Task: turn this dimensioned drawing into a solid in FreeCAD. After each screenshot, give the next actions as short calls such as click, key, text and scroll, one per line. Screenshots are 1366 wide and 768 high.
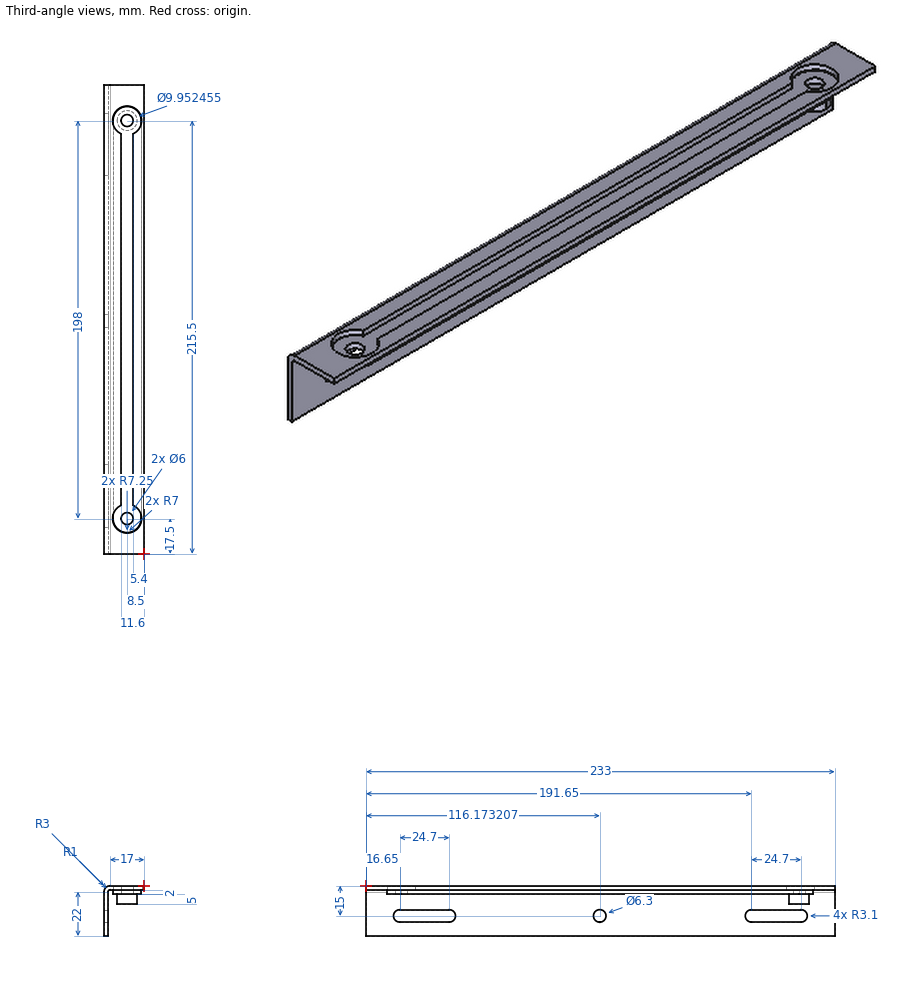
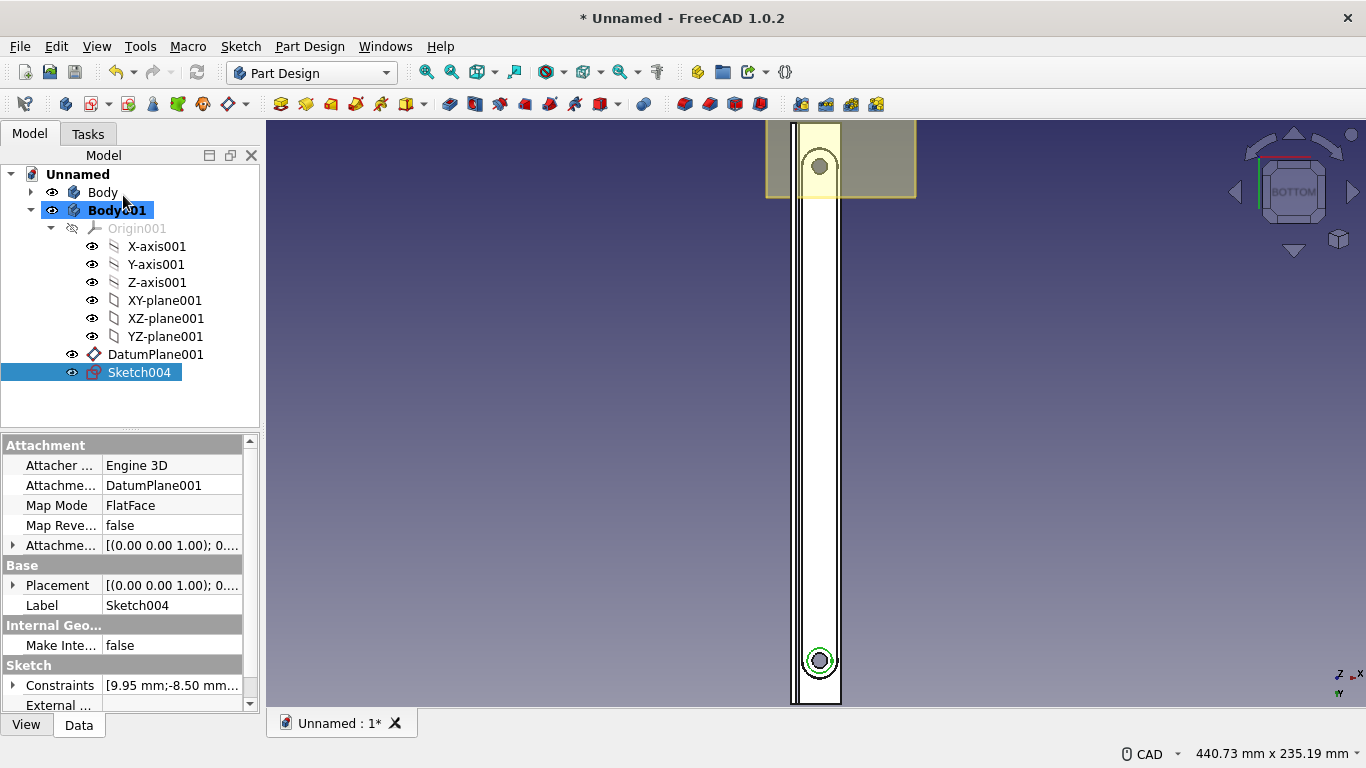
click(281, 104)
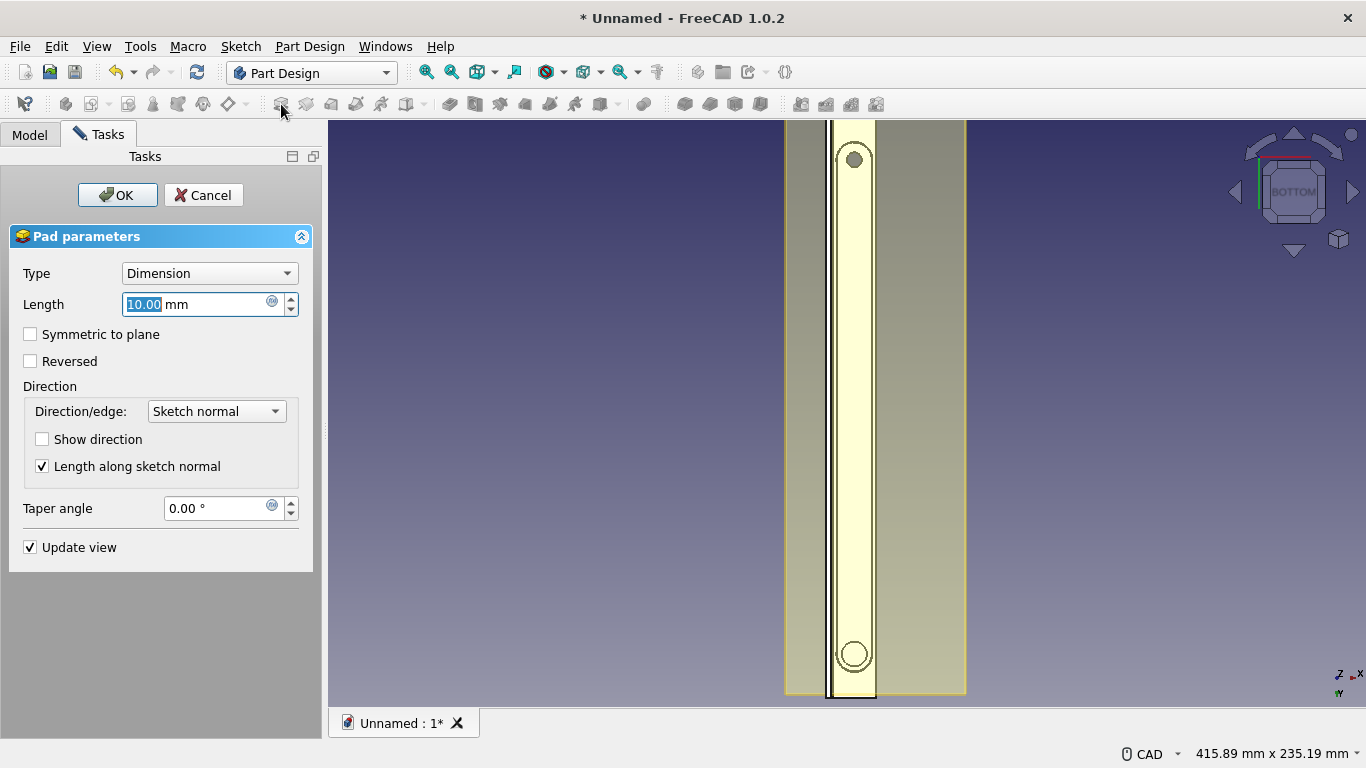
text(5)
key(Tab)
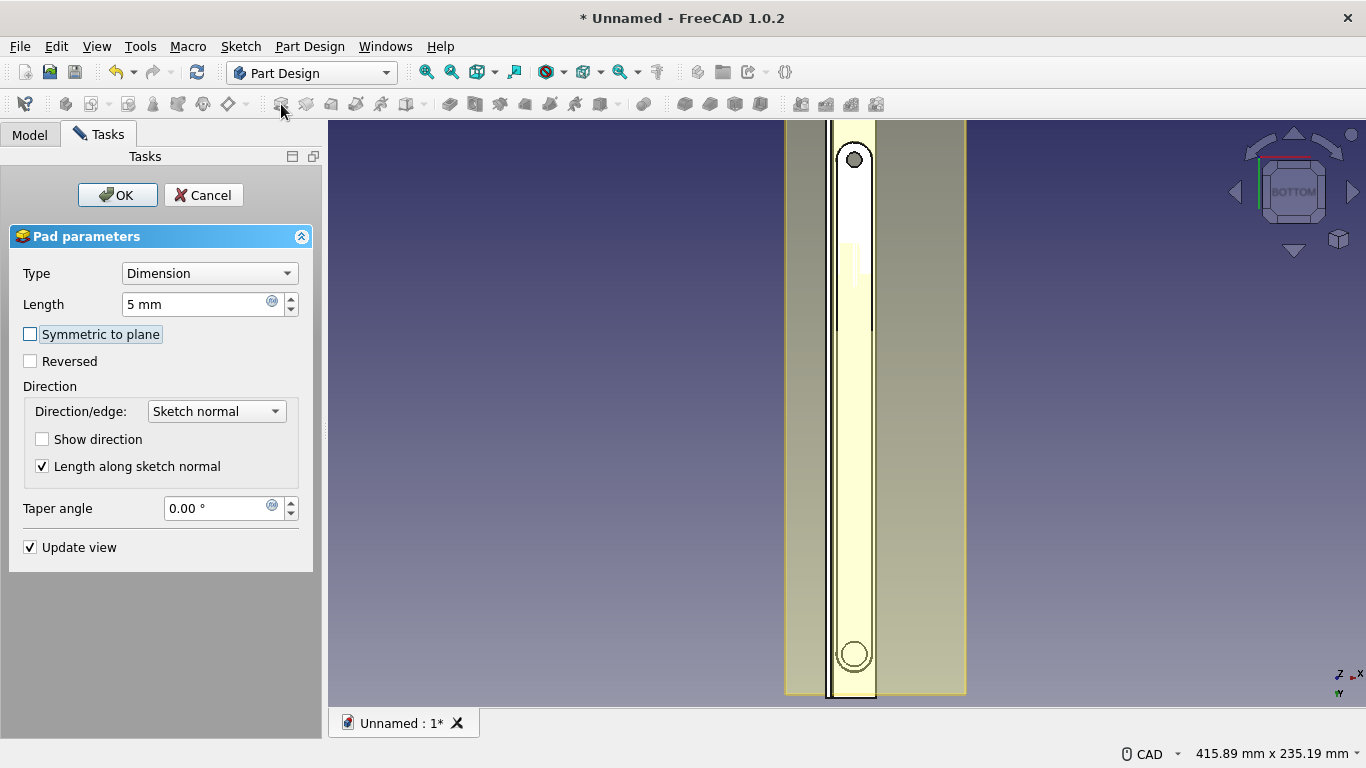
click(31, 361)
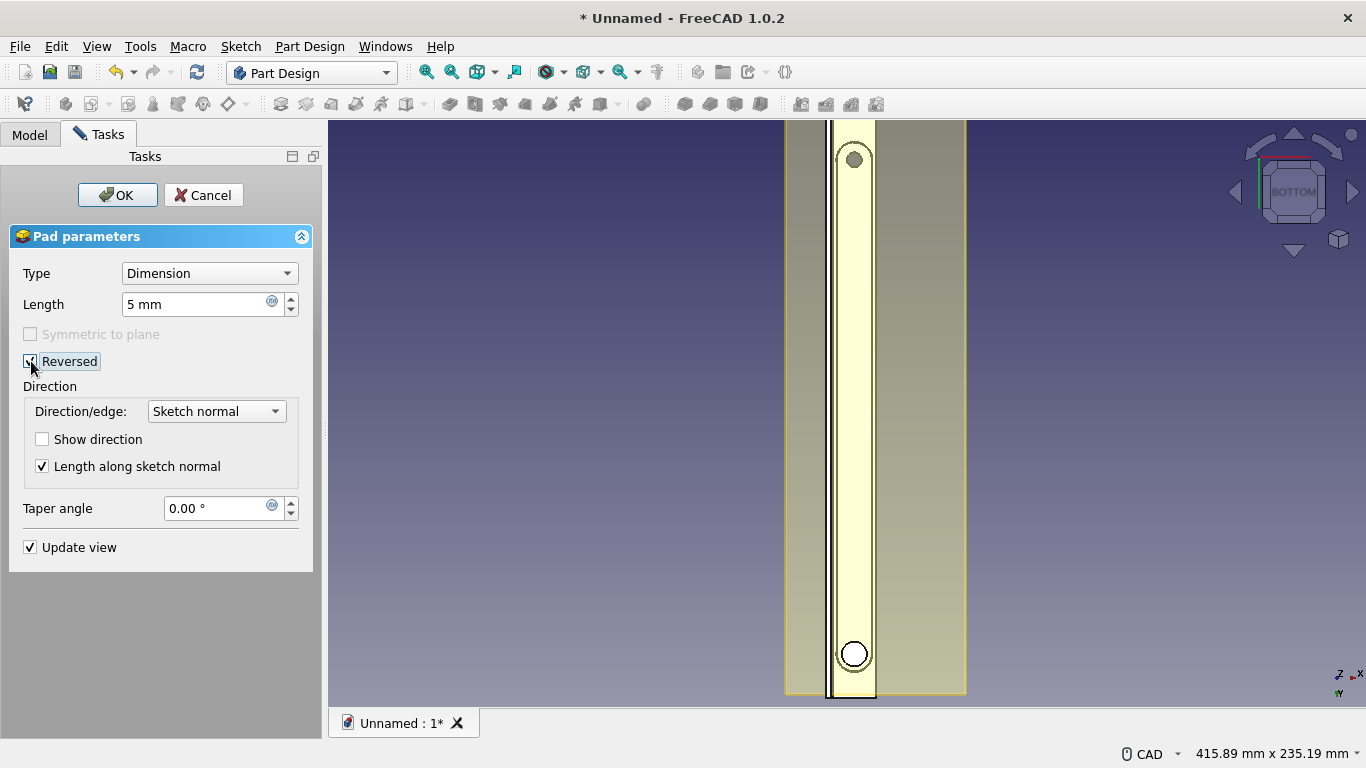
click(118, 195)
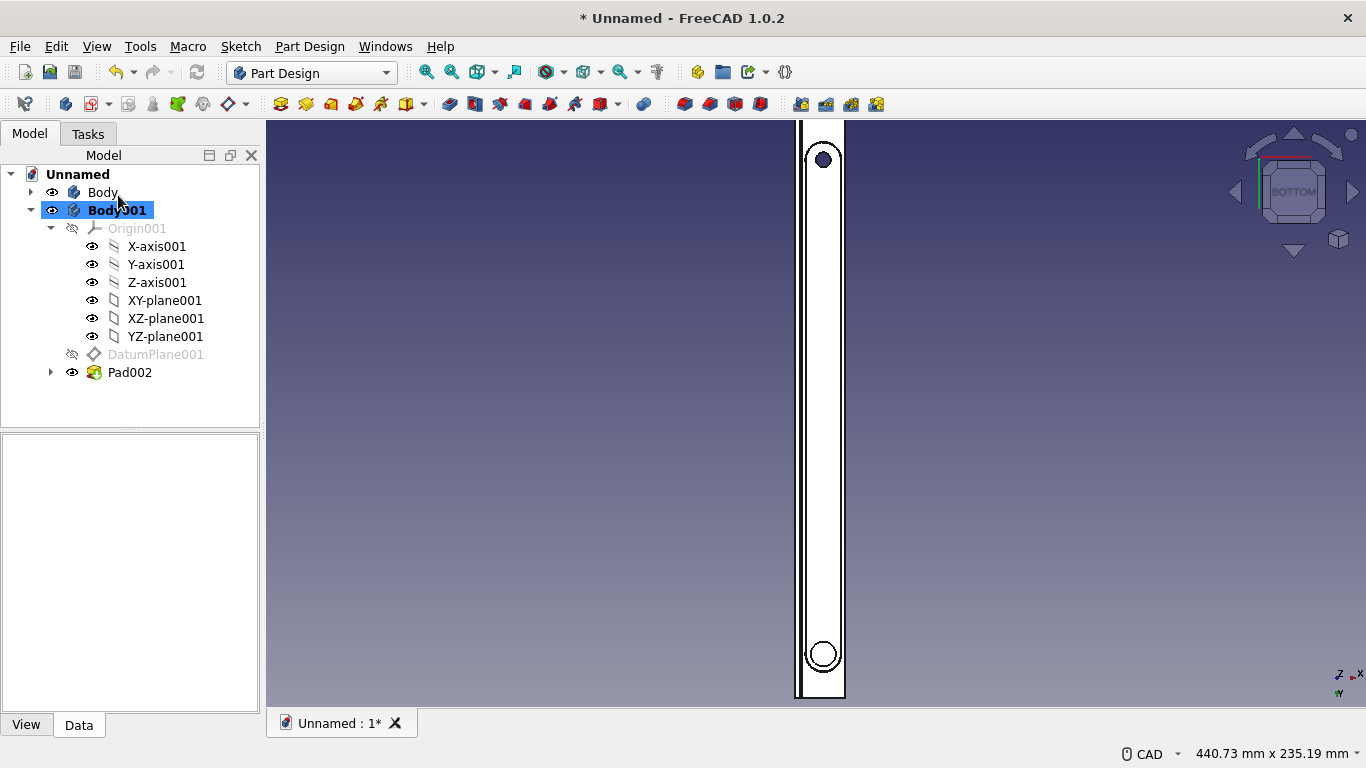
key(0)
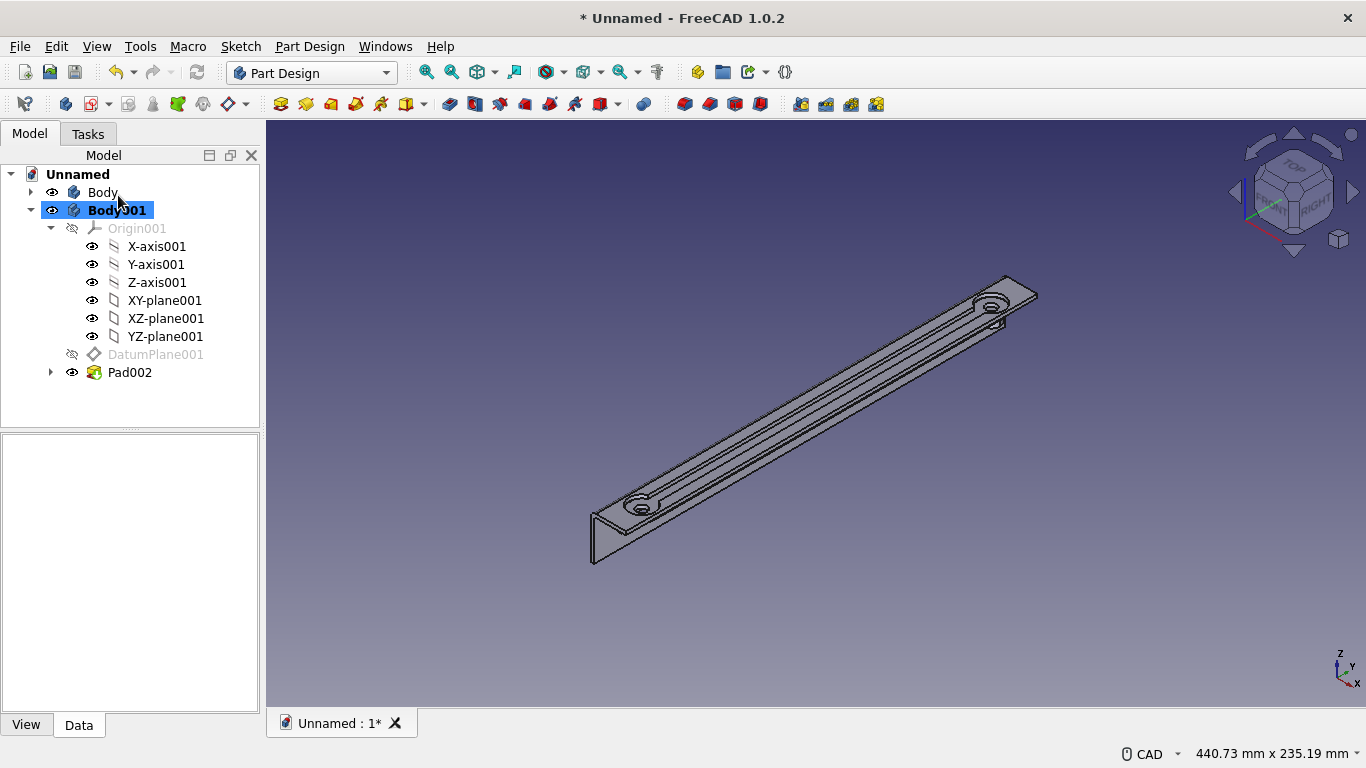
click(427, 72)